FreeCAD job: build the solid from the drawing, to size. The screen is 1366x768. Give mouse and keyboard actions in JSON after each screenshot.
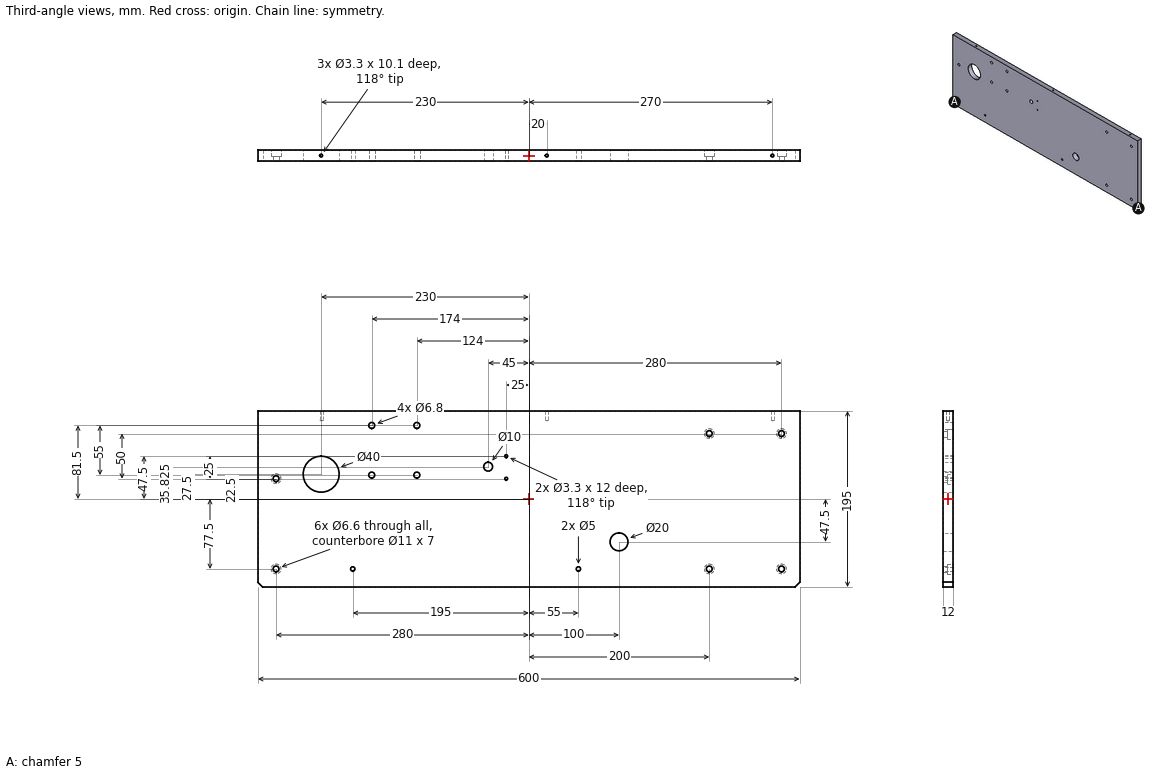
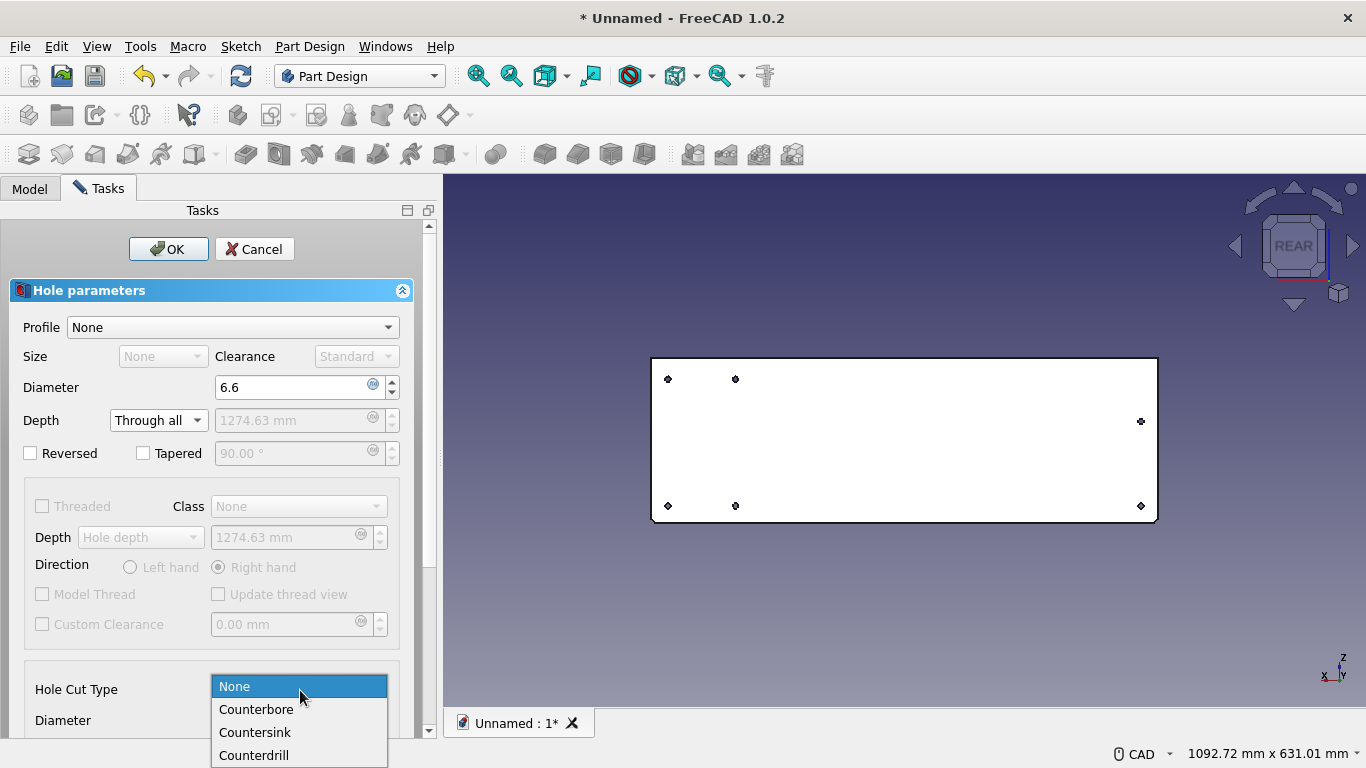
{"action": "left_click", "coordinate": [298, 710]}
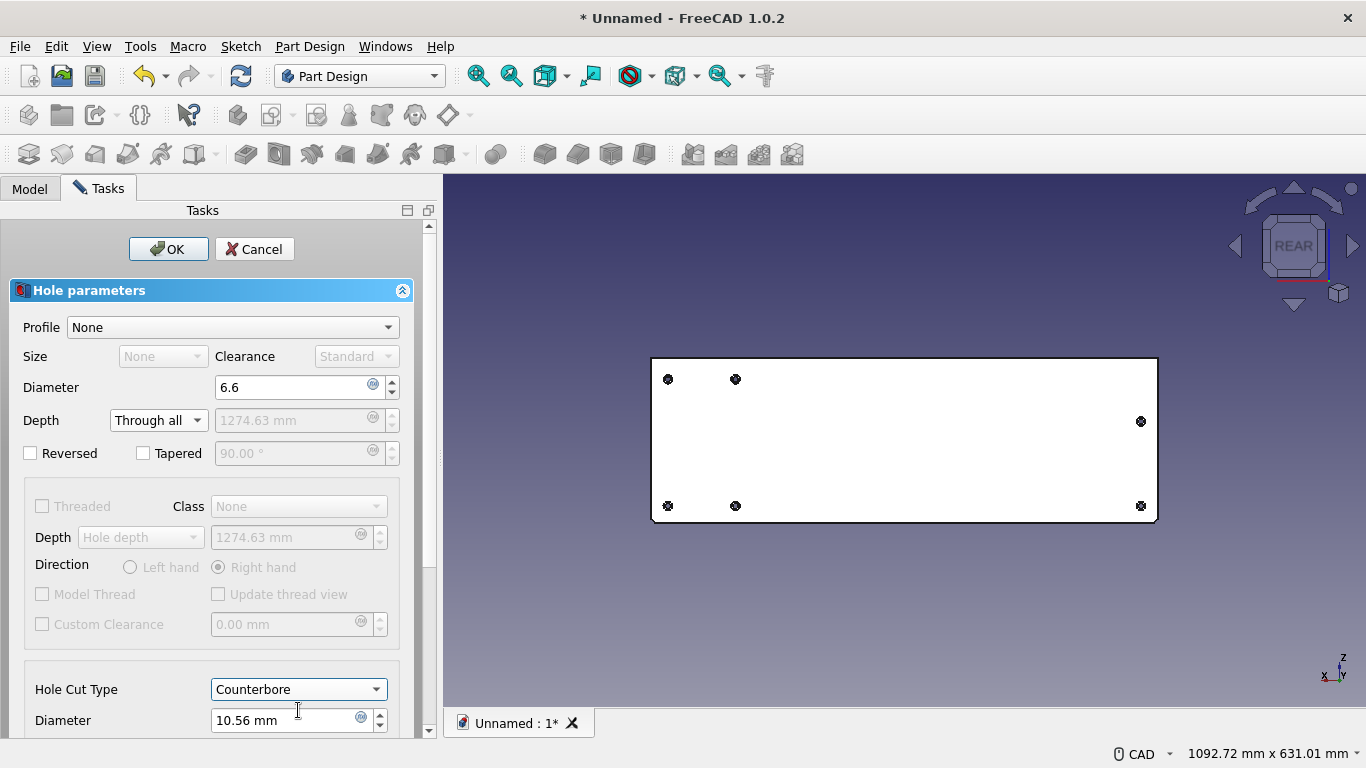
{"action": "triple_click", "coordinate": [292, 720]}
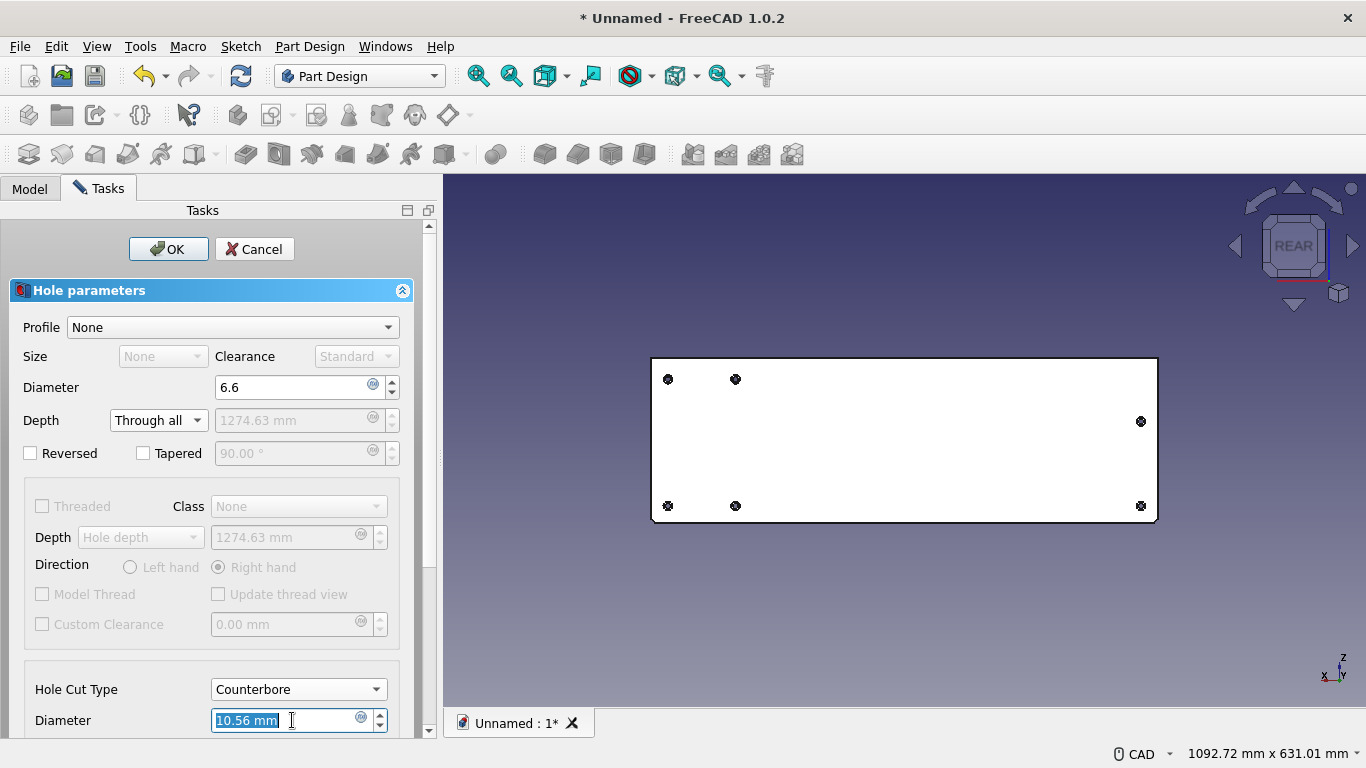
{"action": "type", "text": "11"}
{"action": "key", "text": "Tab"}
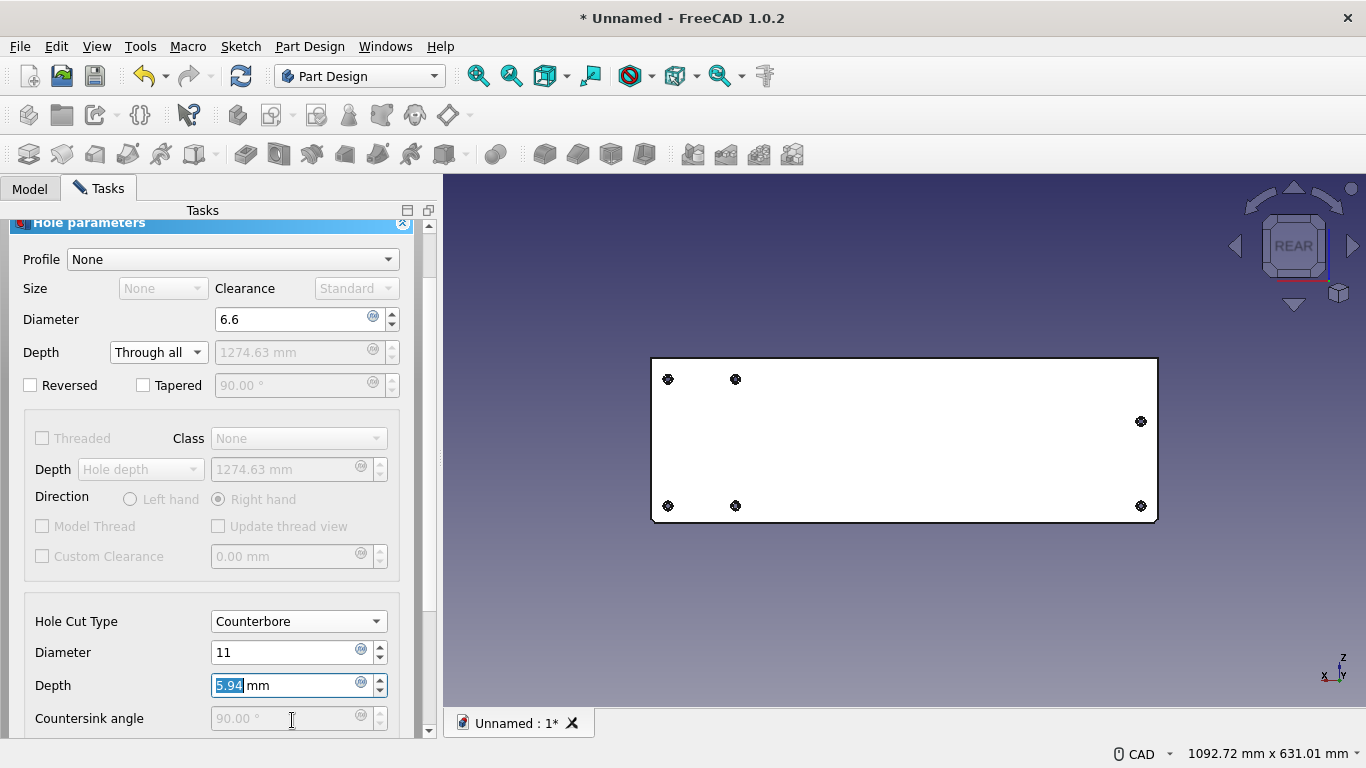
{"action": "type", "text": "7"}
{"action": "key", "text": "Tab"}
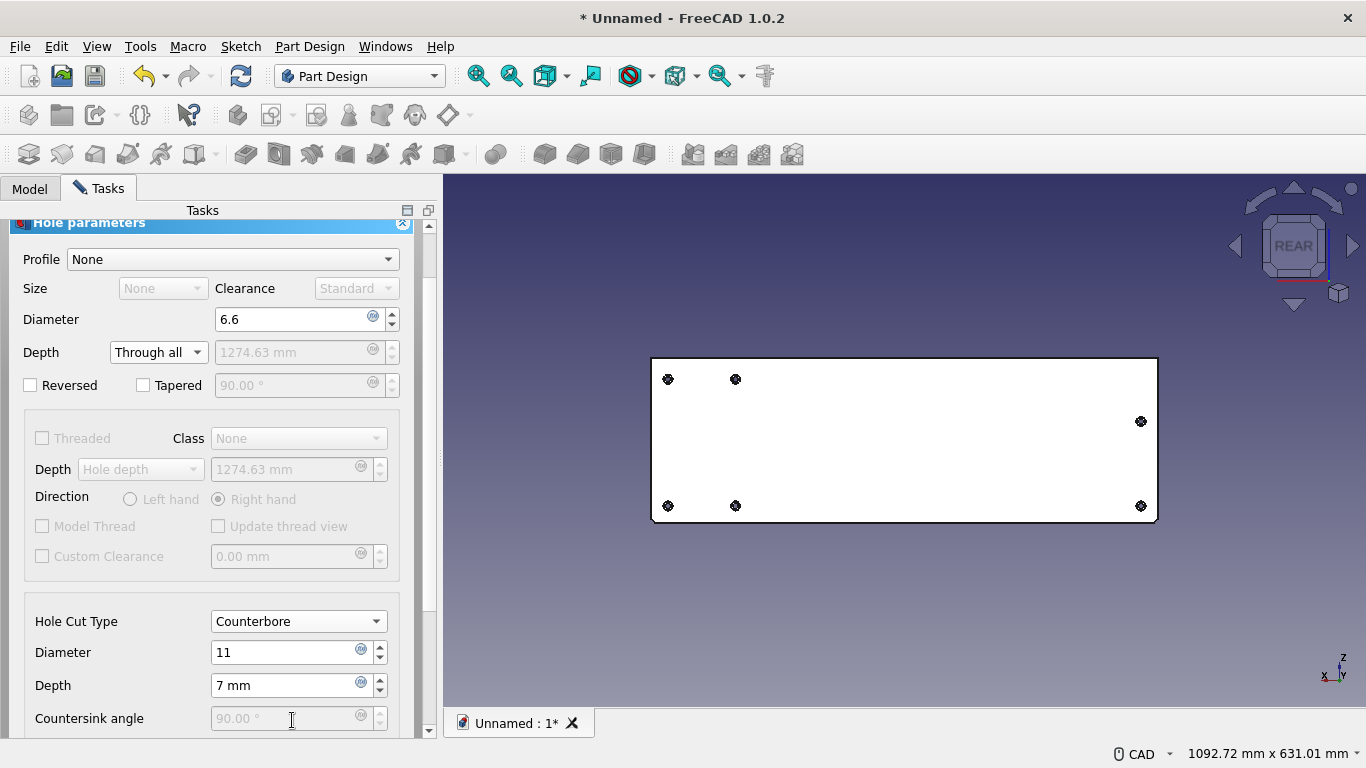
{"action": "scroll", "coordinate": [429, 479], "scroll_direction": "up", "scroll_amount": 2}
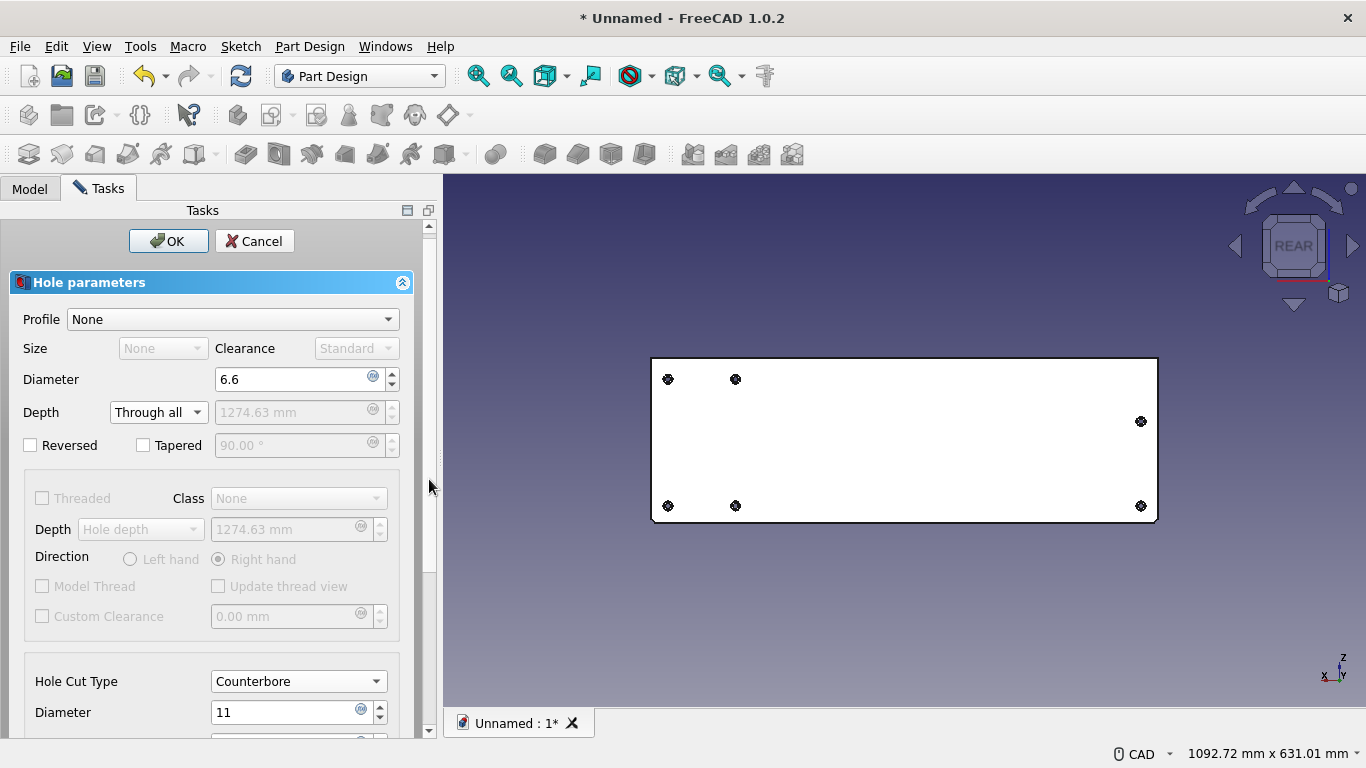
{"action": "left_click", "coordinate": [169, 249]}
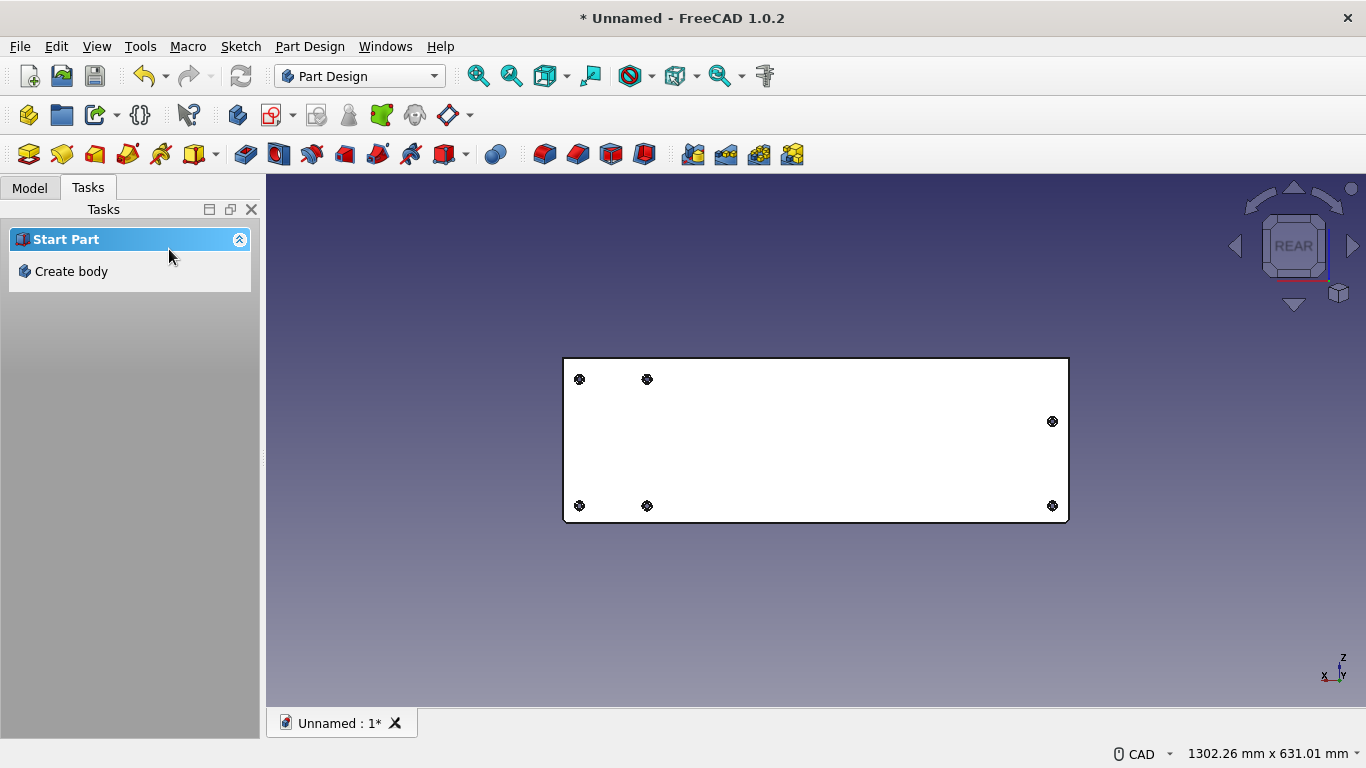
{"action": "key", "text": "0"}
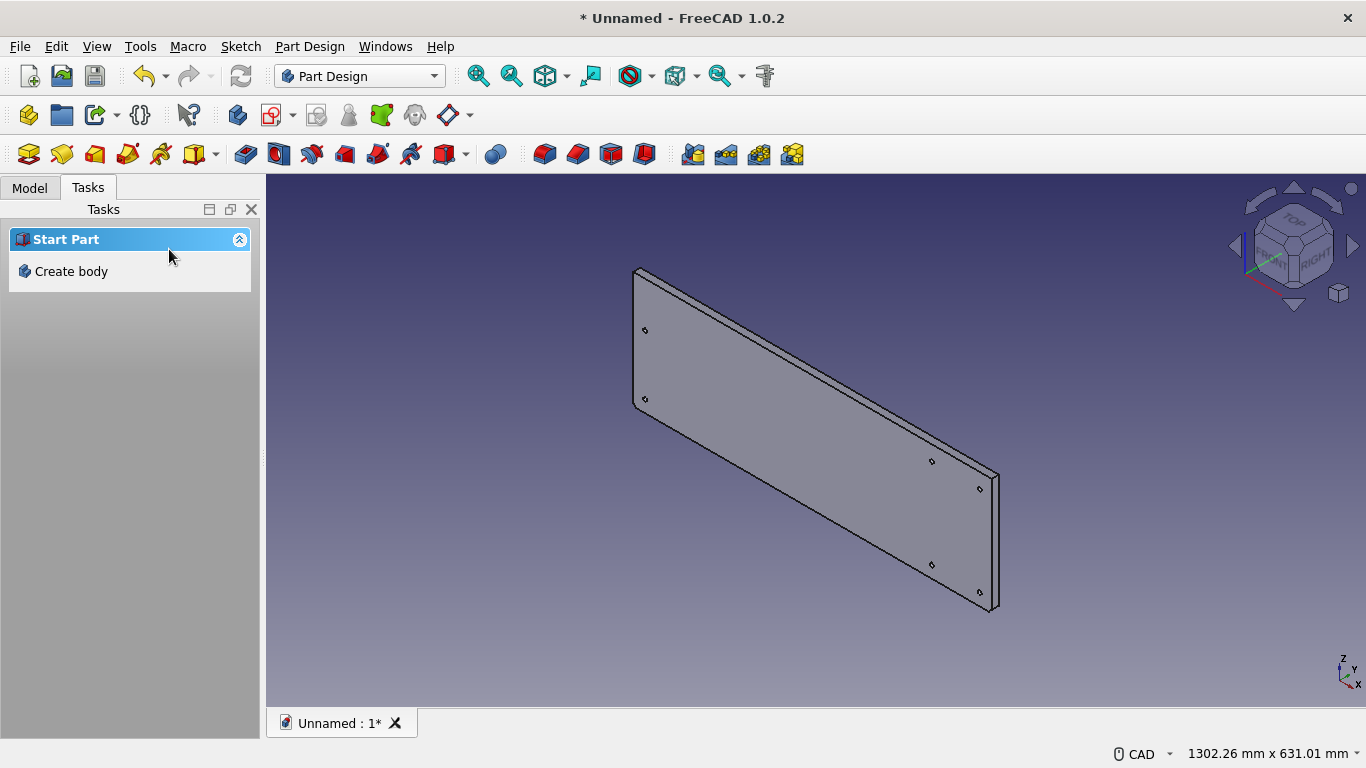
{"action": "scroll", "coordinate": [970, 461], "scroll_direction": "up", "scroll_amount": 5}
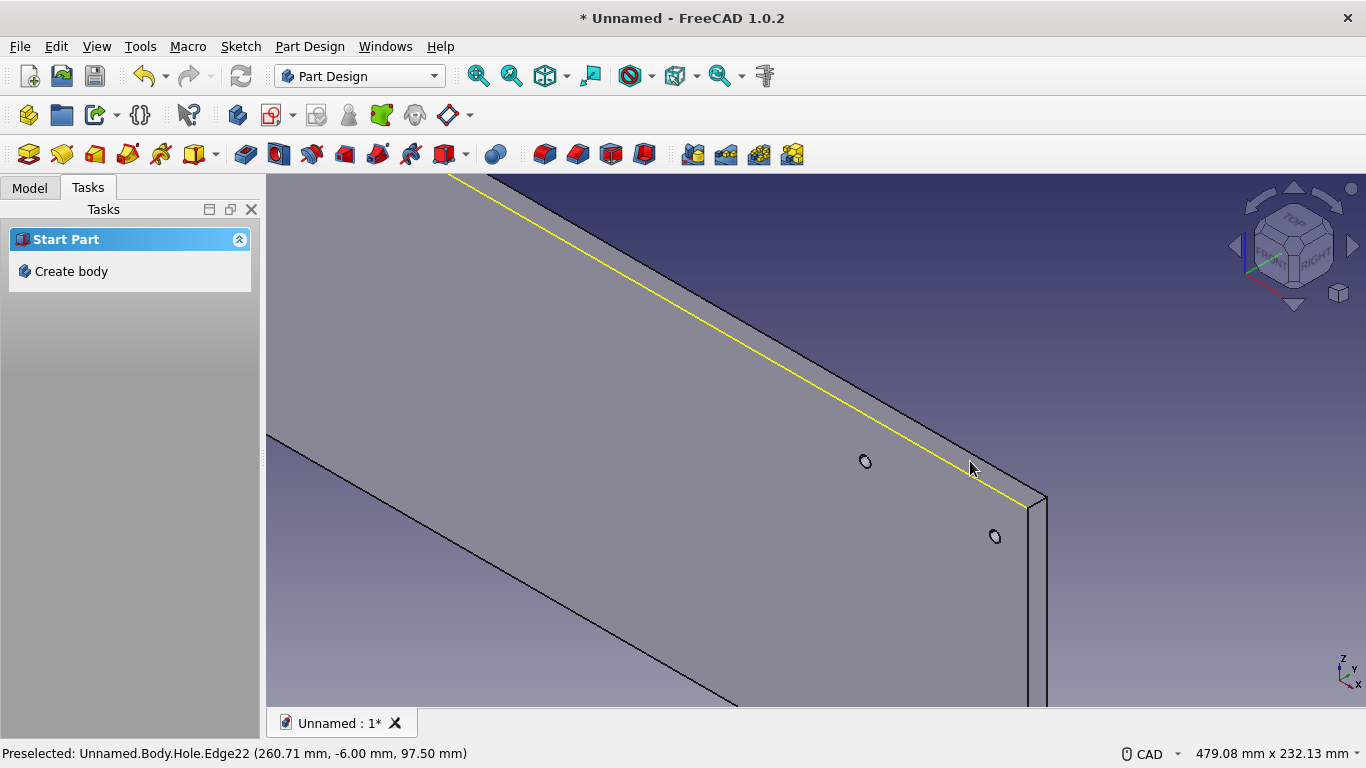
{"action": "left_click", "coordinate": [968, 462]}